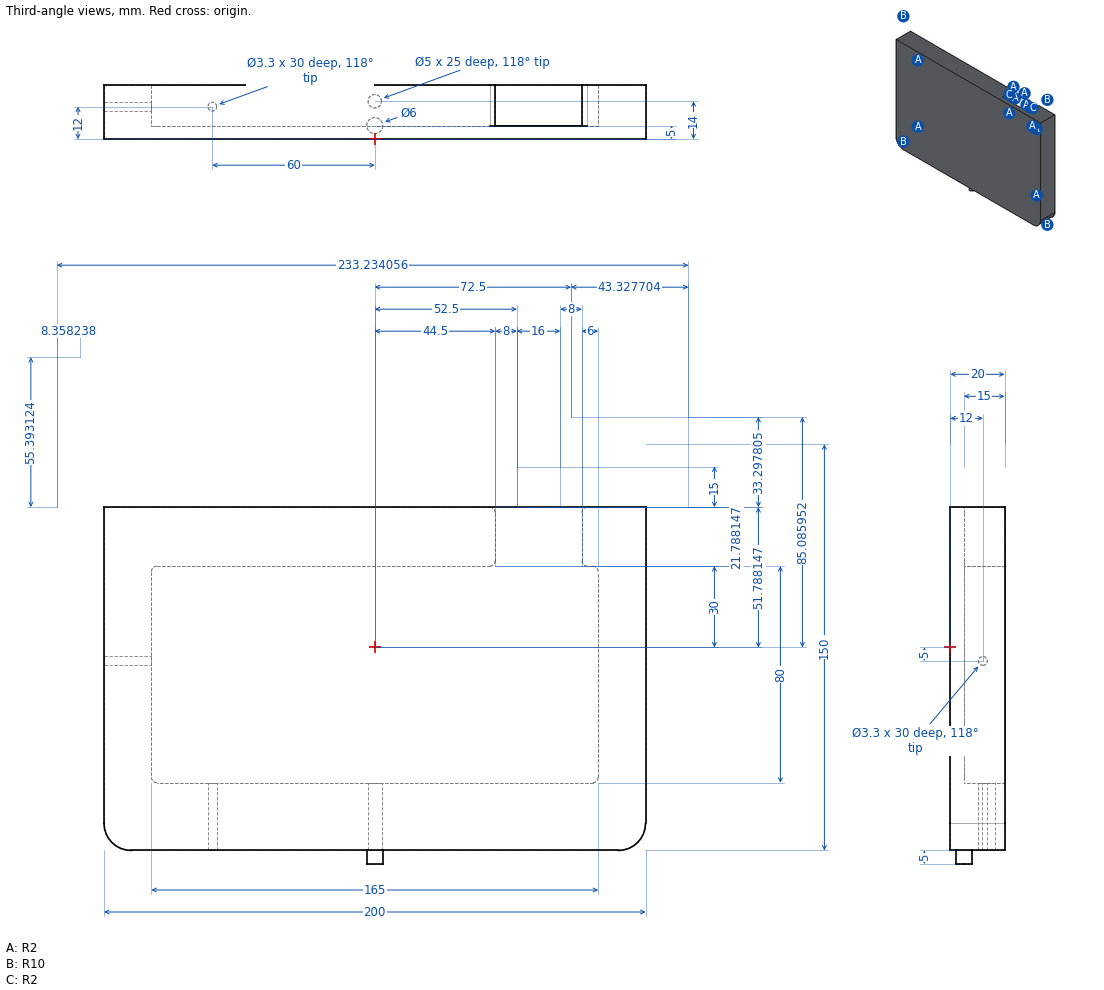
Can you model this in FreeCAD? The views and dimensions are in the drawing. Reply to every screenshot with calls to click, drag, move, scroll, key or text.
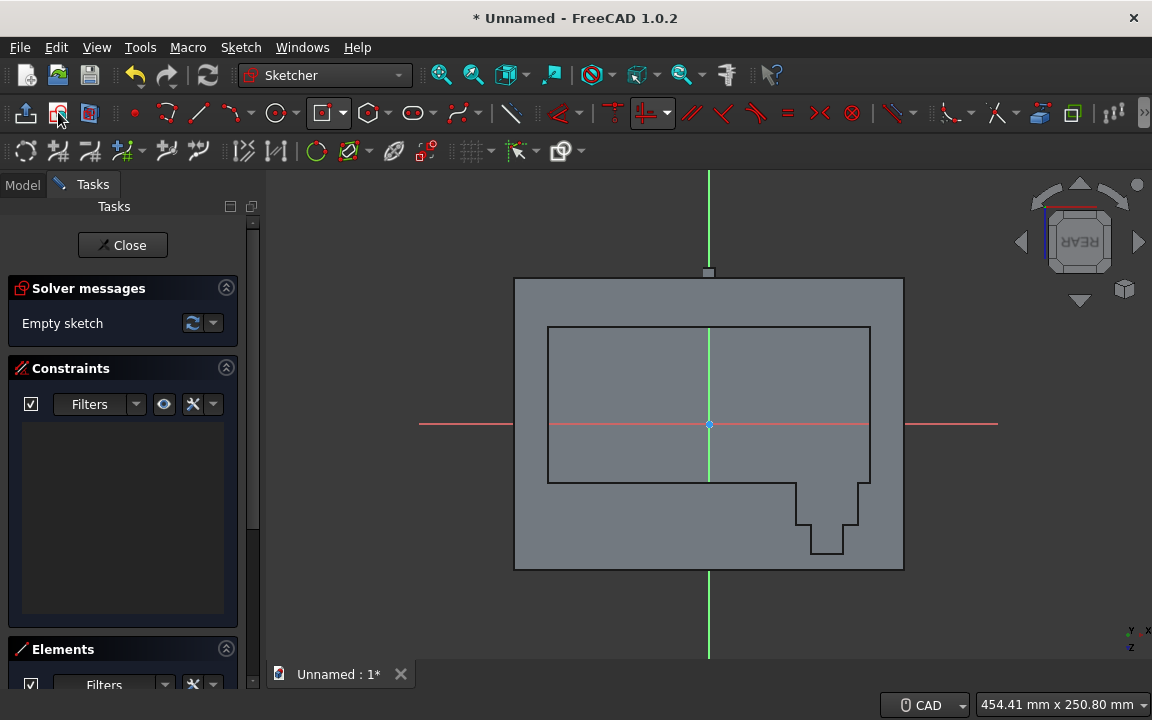
click(90, 114)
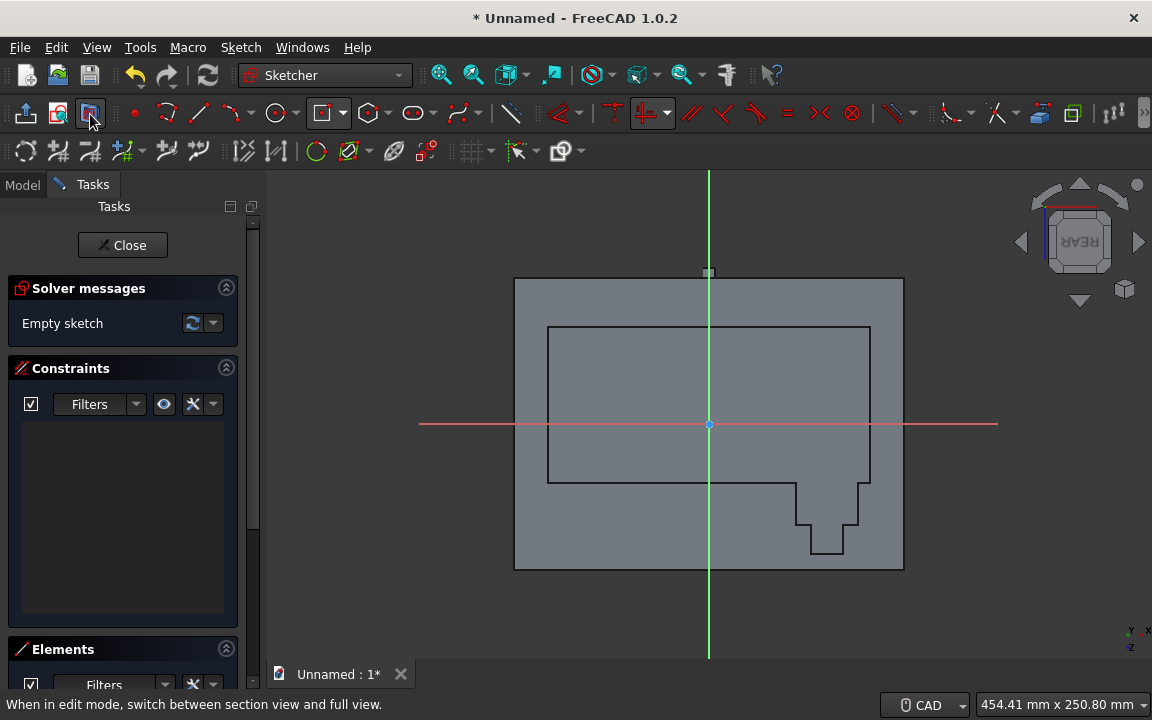
scroll(846, 552, up, 12)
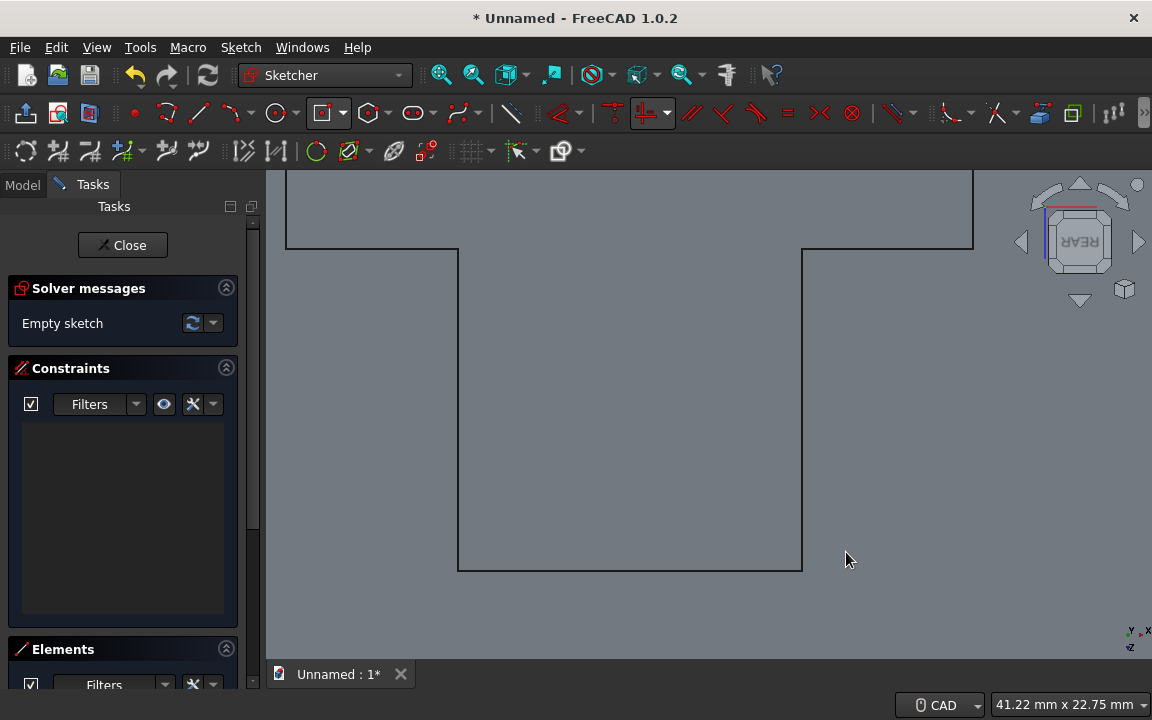
key(g)
key(r)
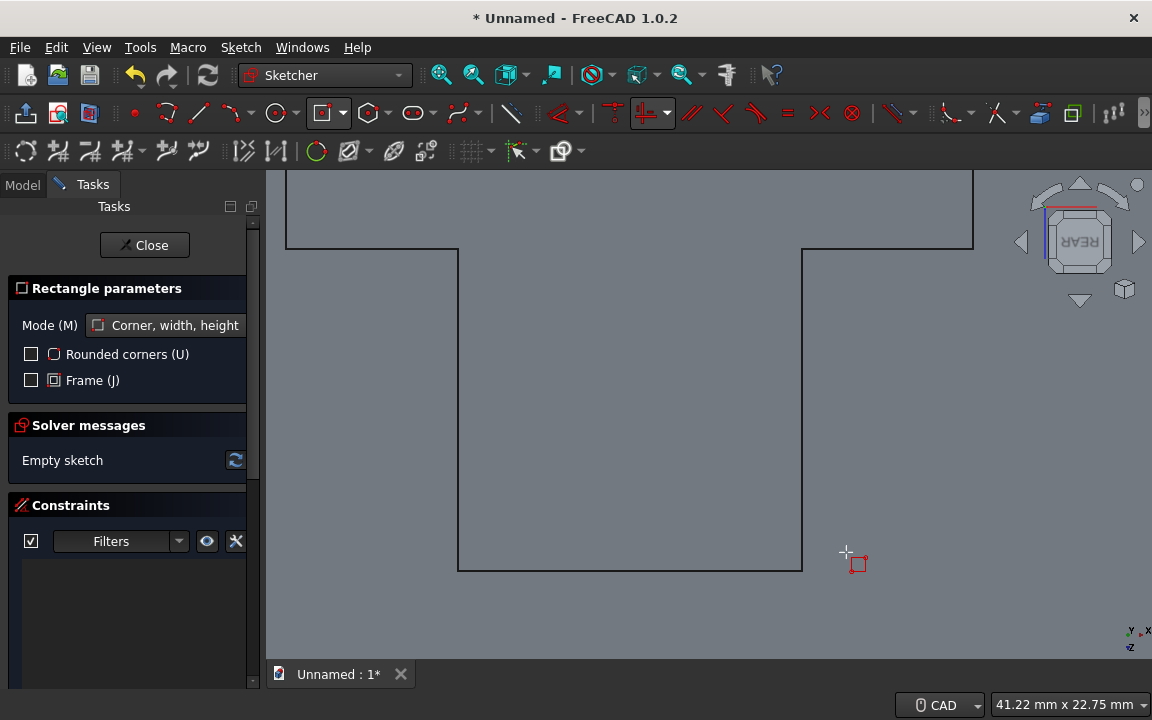
click(458, 249)
click(802, 571)
key(Escape)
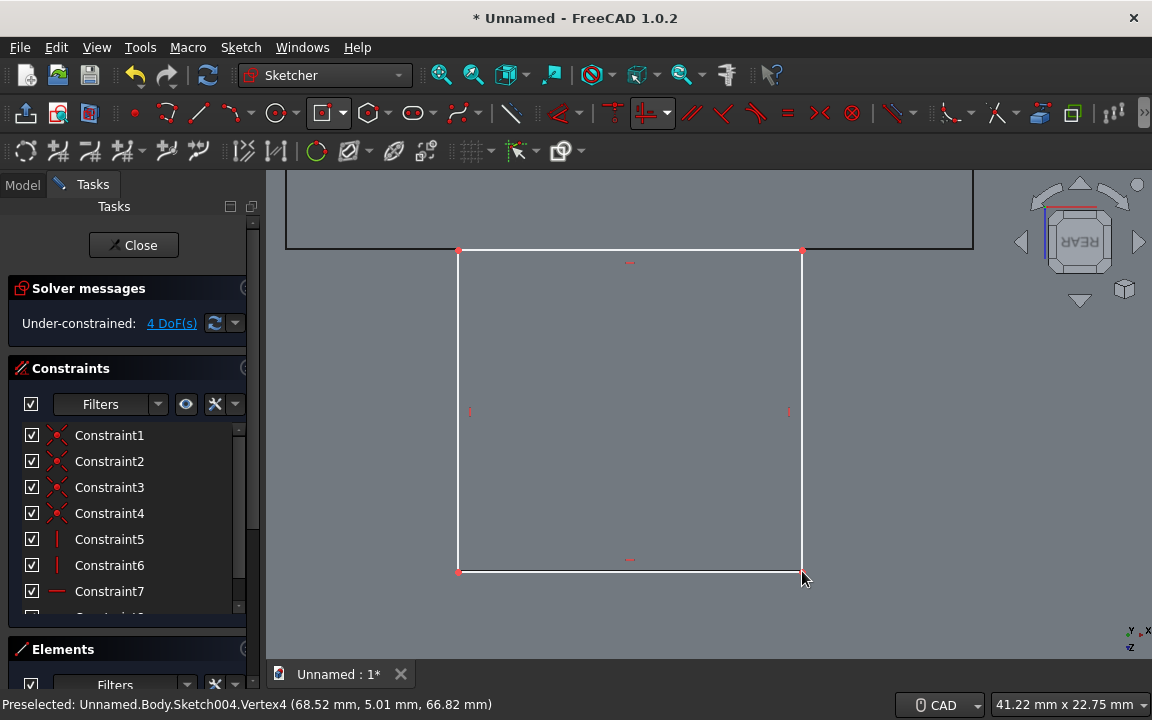
key(d)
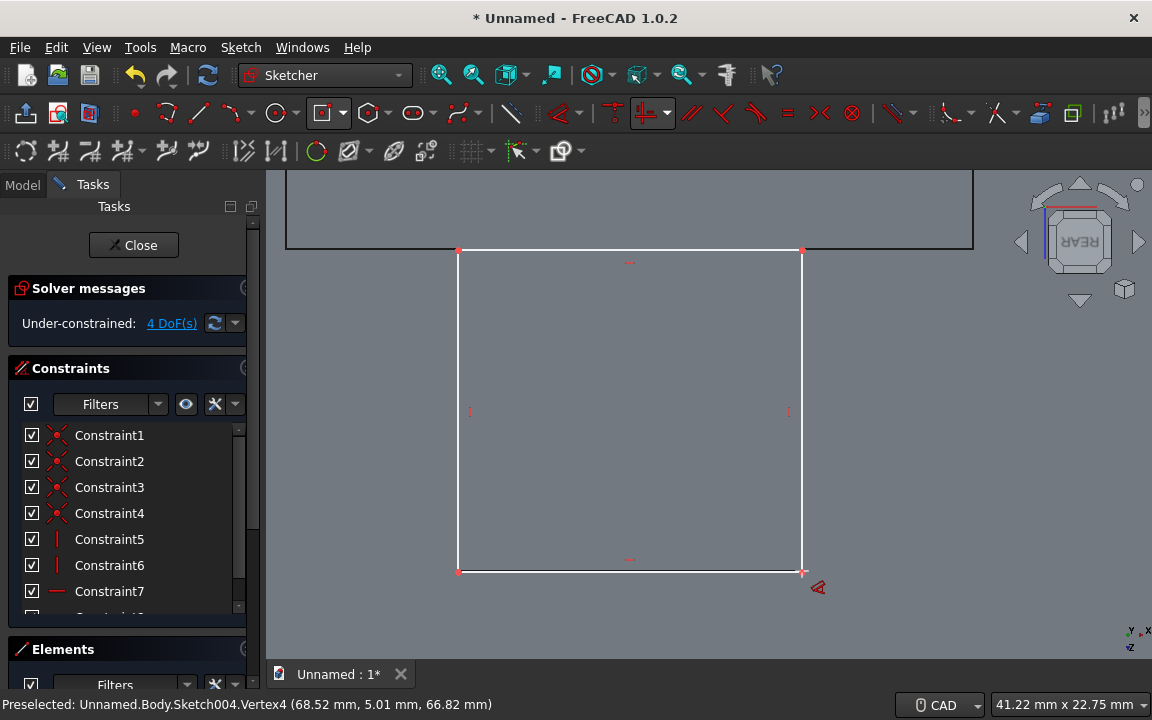
click(458, 347)
click(424, 411)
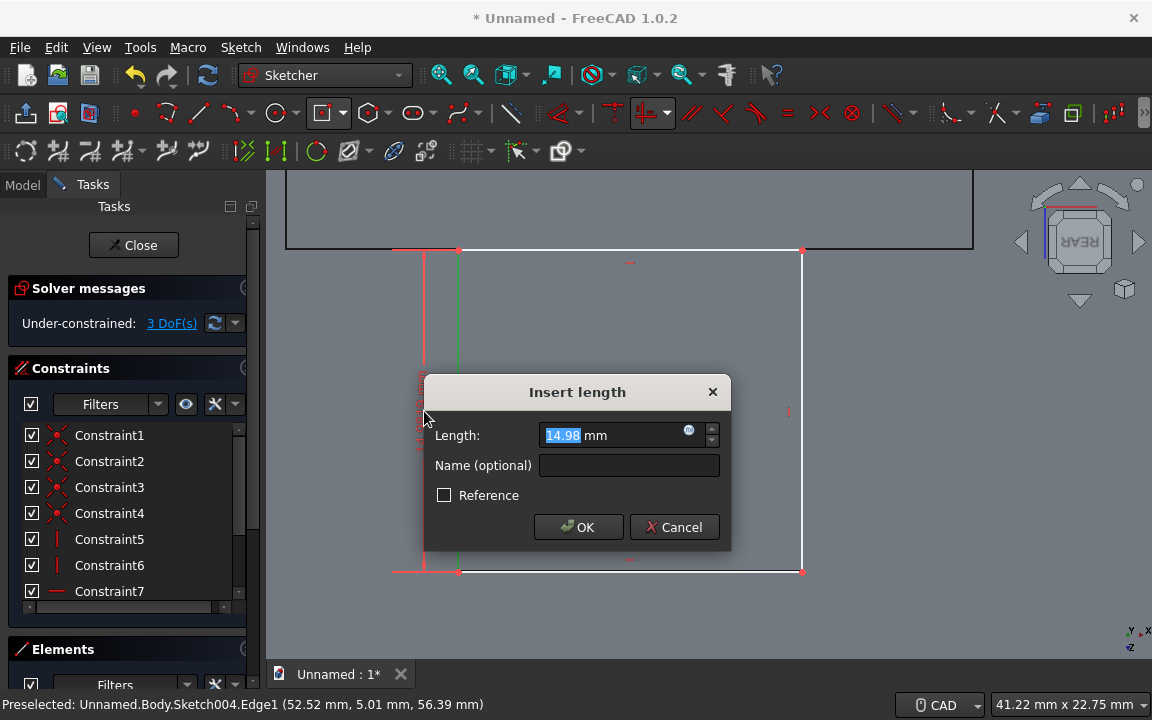
text(15)
key(Return)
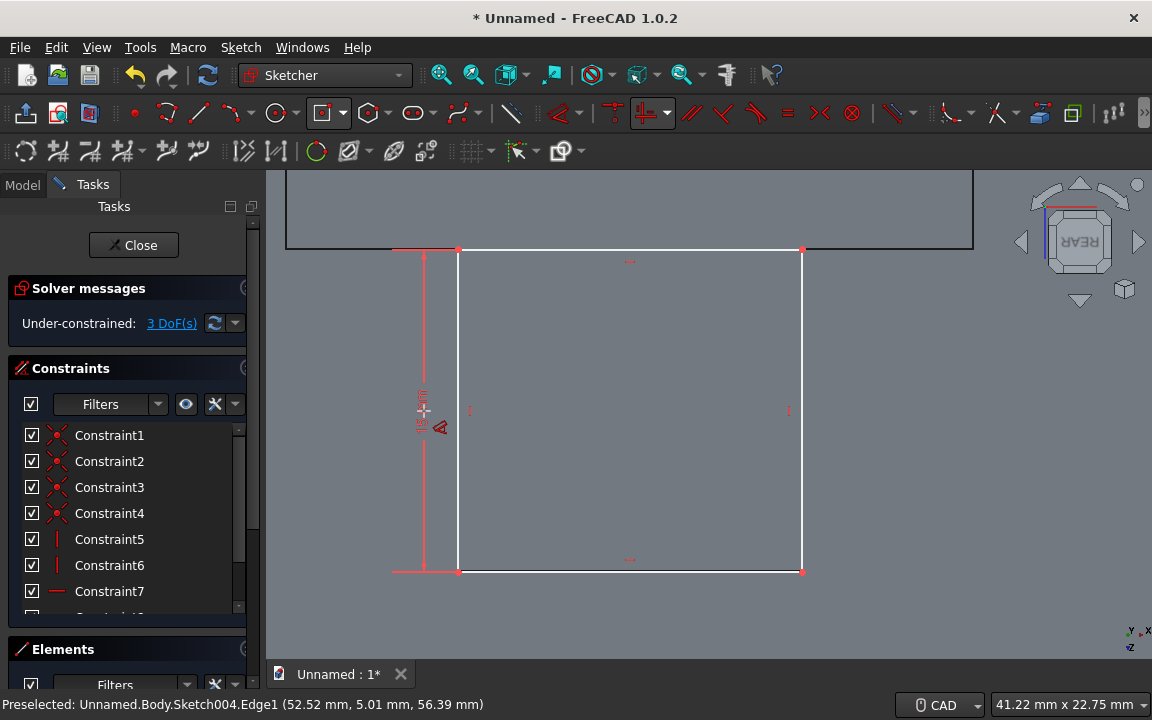
click(561, 572)
click(630, 606)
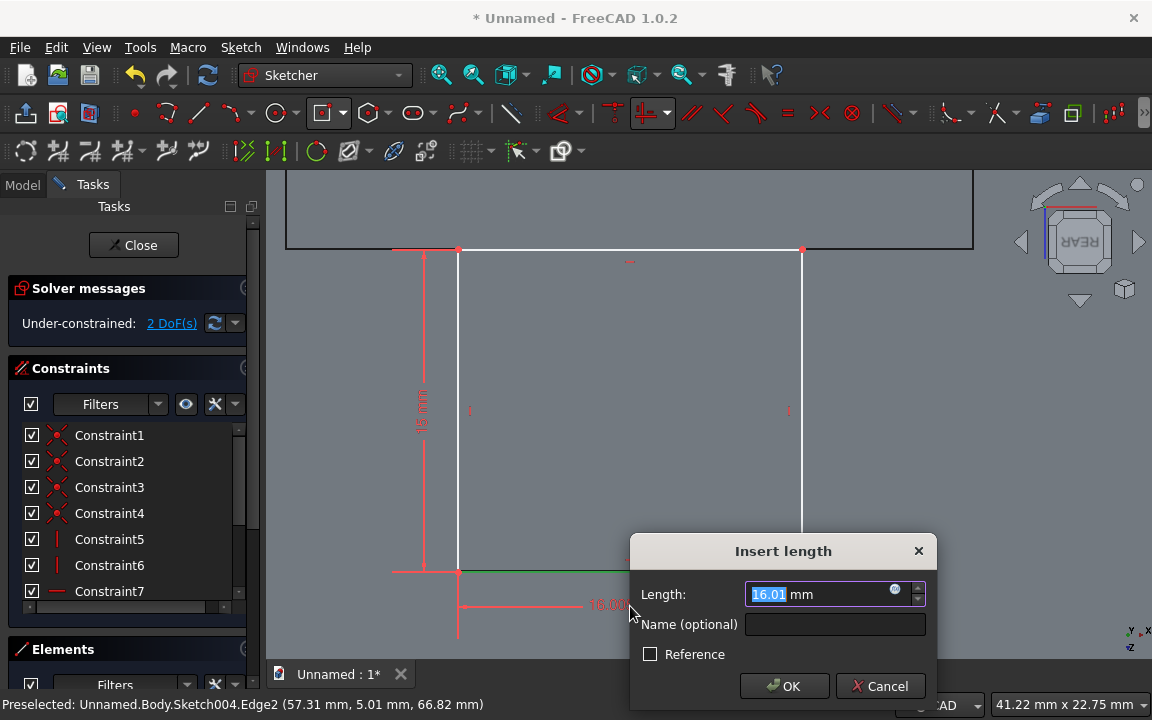
text(16)
key(Return)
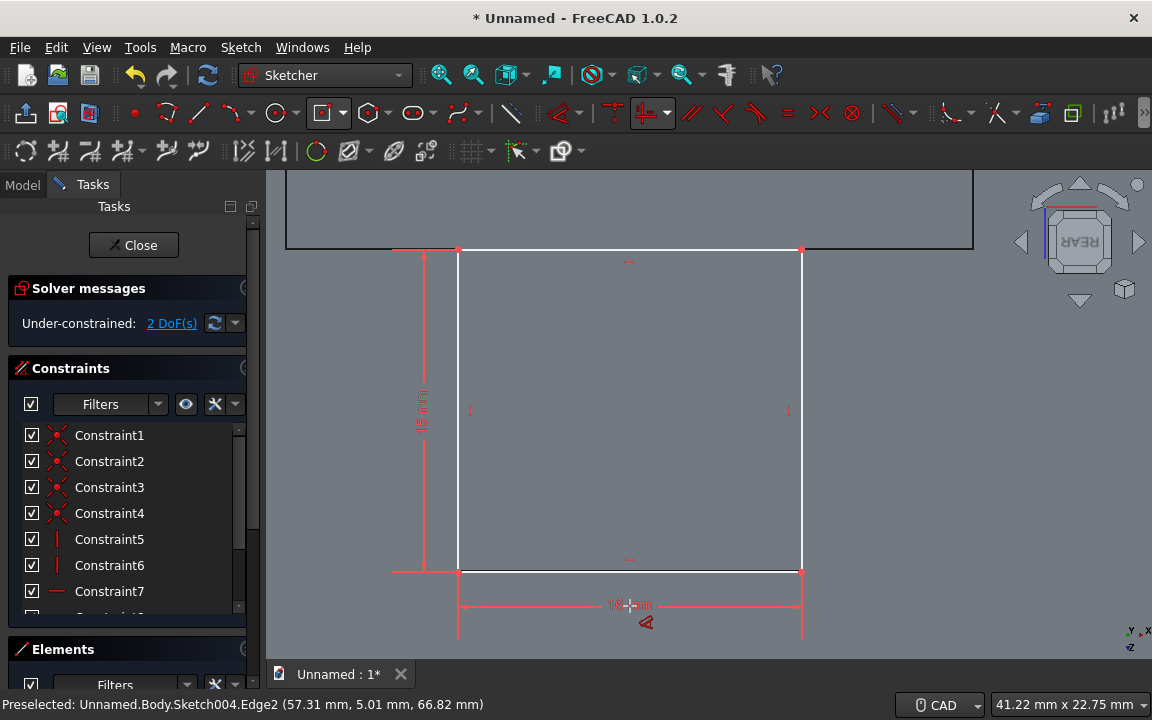
click(458, 250)
click(376, 284)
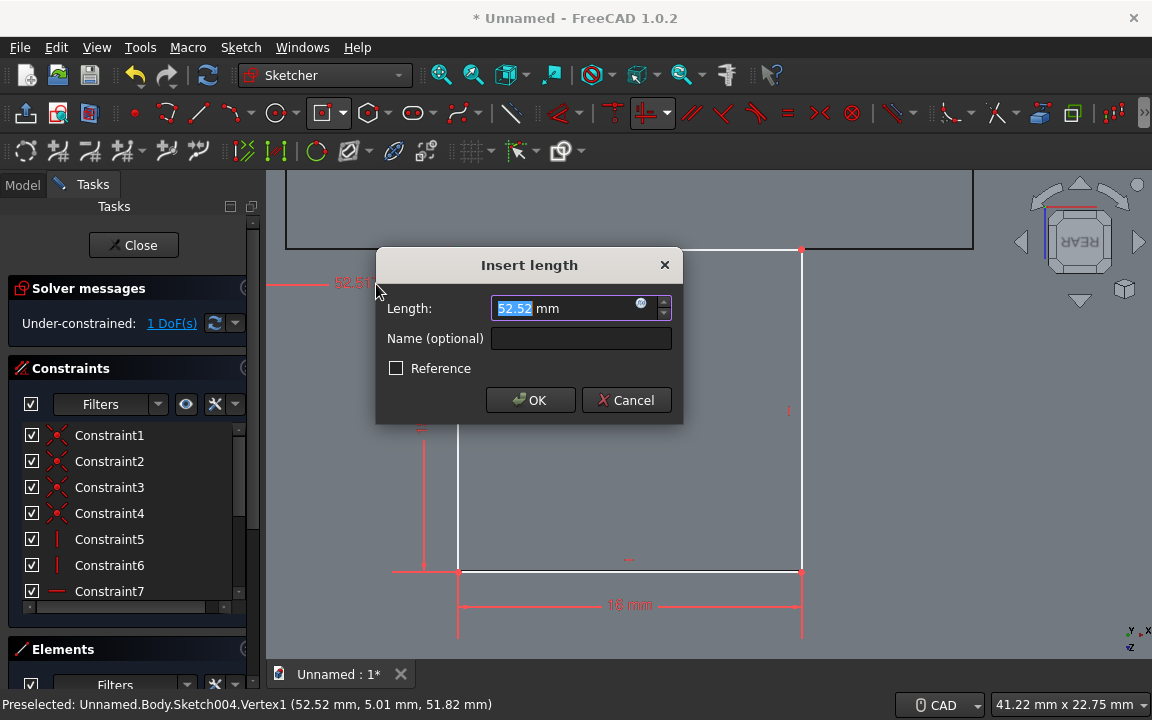
text(52.5)
key(Return)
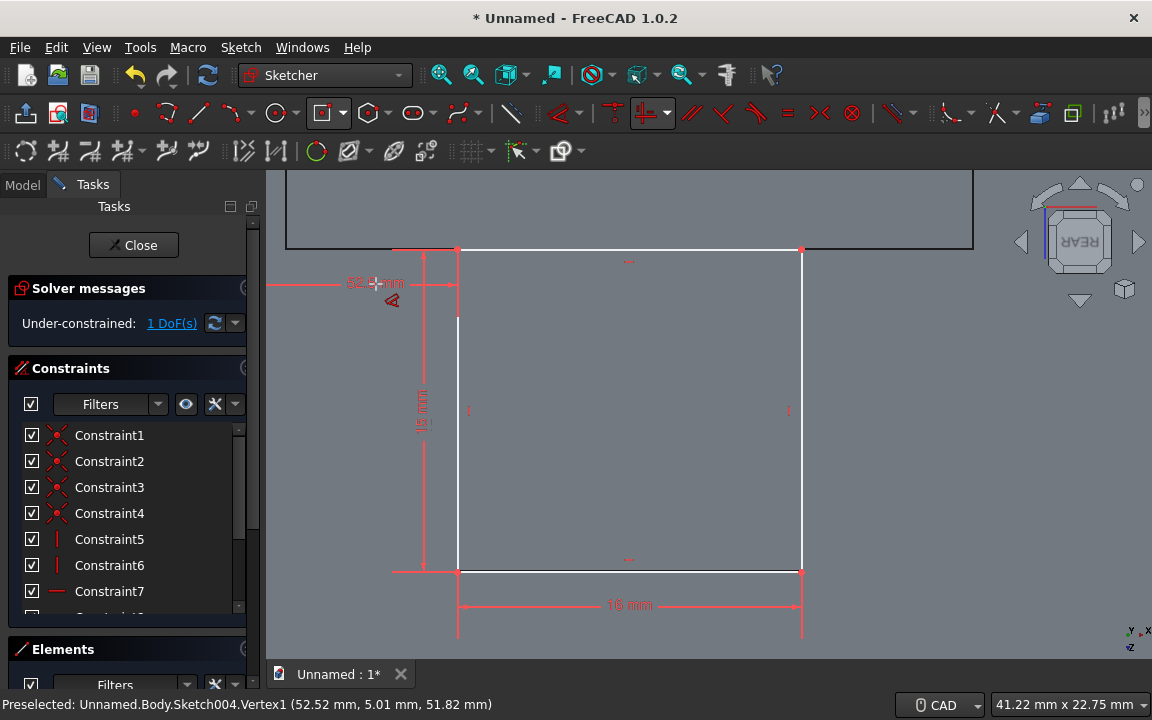
click(458, 250)
click(492, 224)